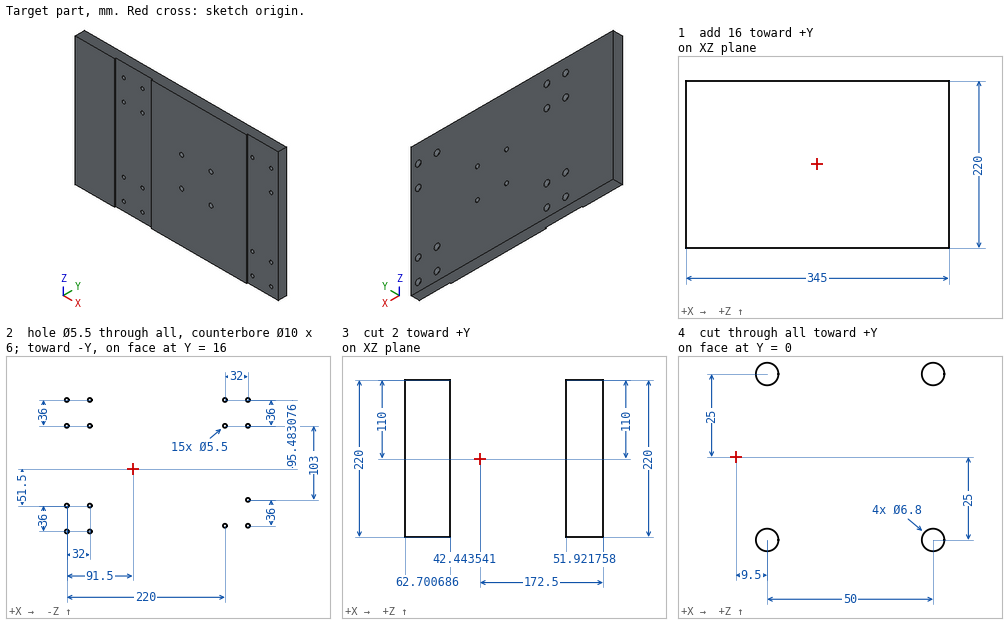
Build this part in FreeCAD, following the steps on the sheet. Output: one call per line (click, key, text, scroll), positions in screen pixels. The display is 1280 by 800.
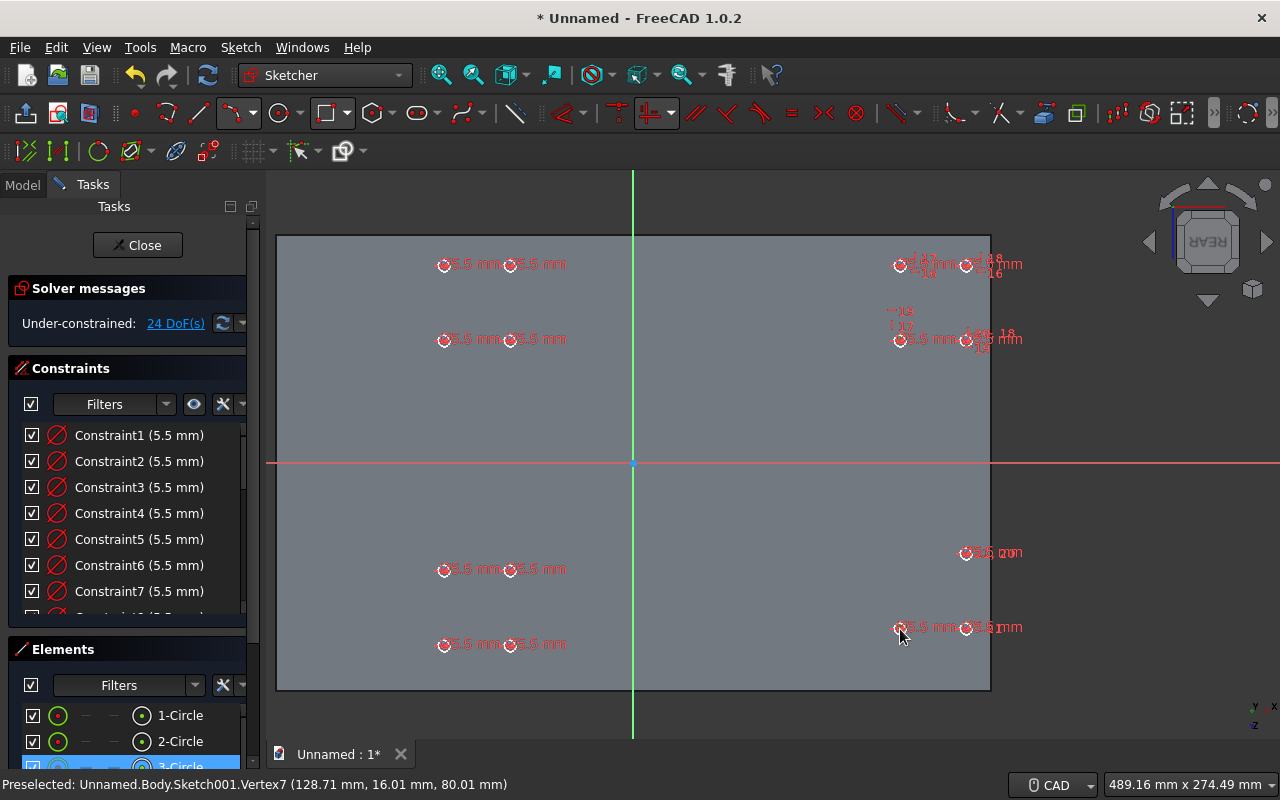
key(v)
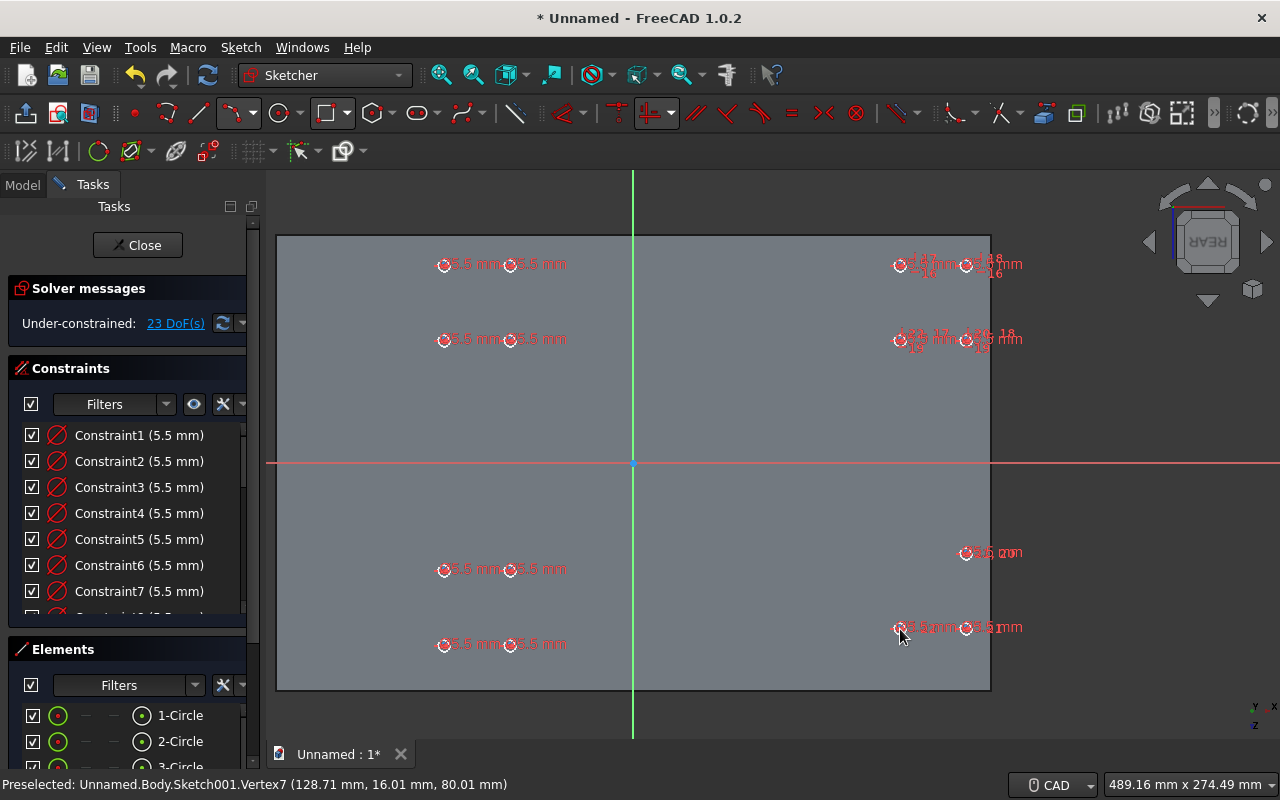
click(966, 629)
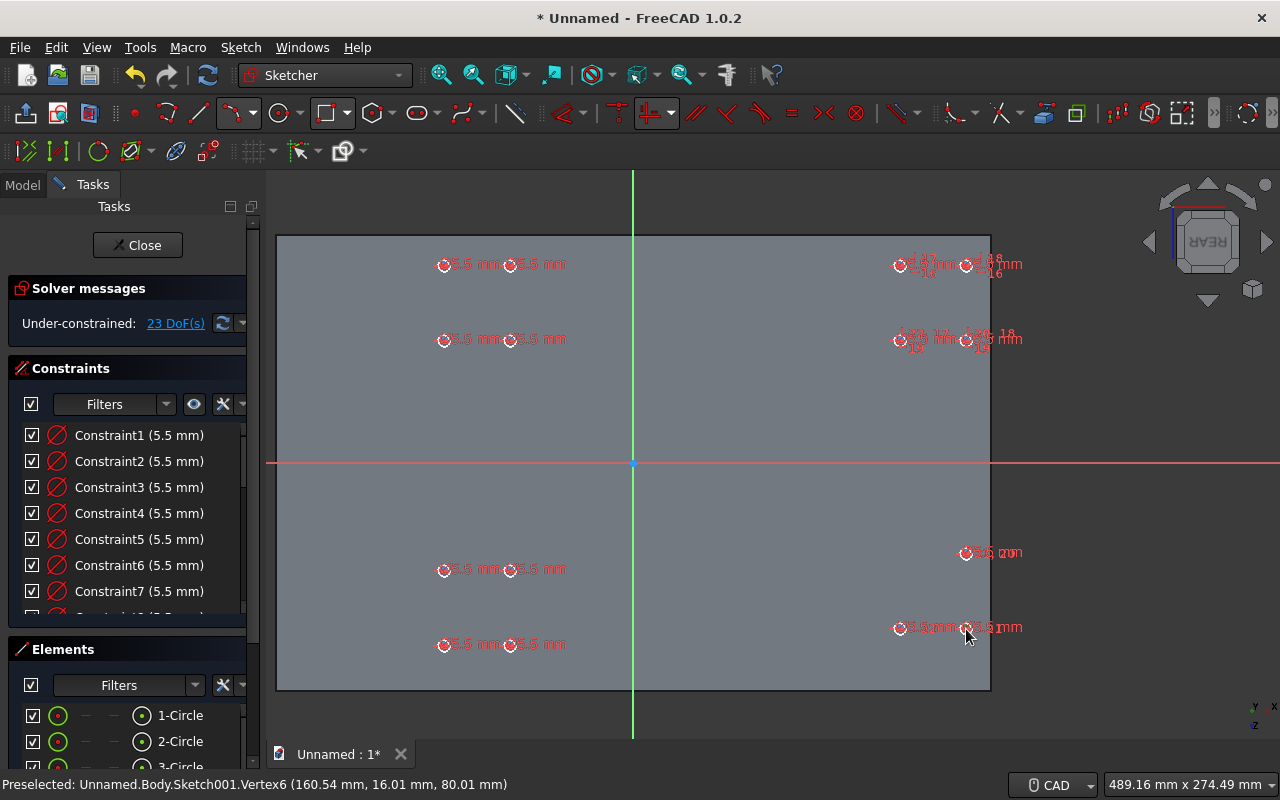
click(900, 629)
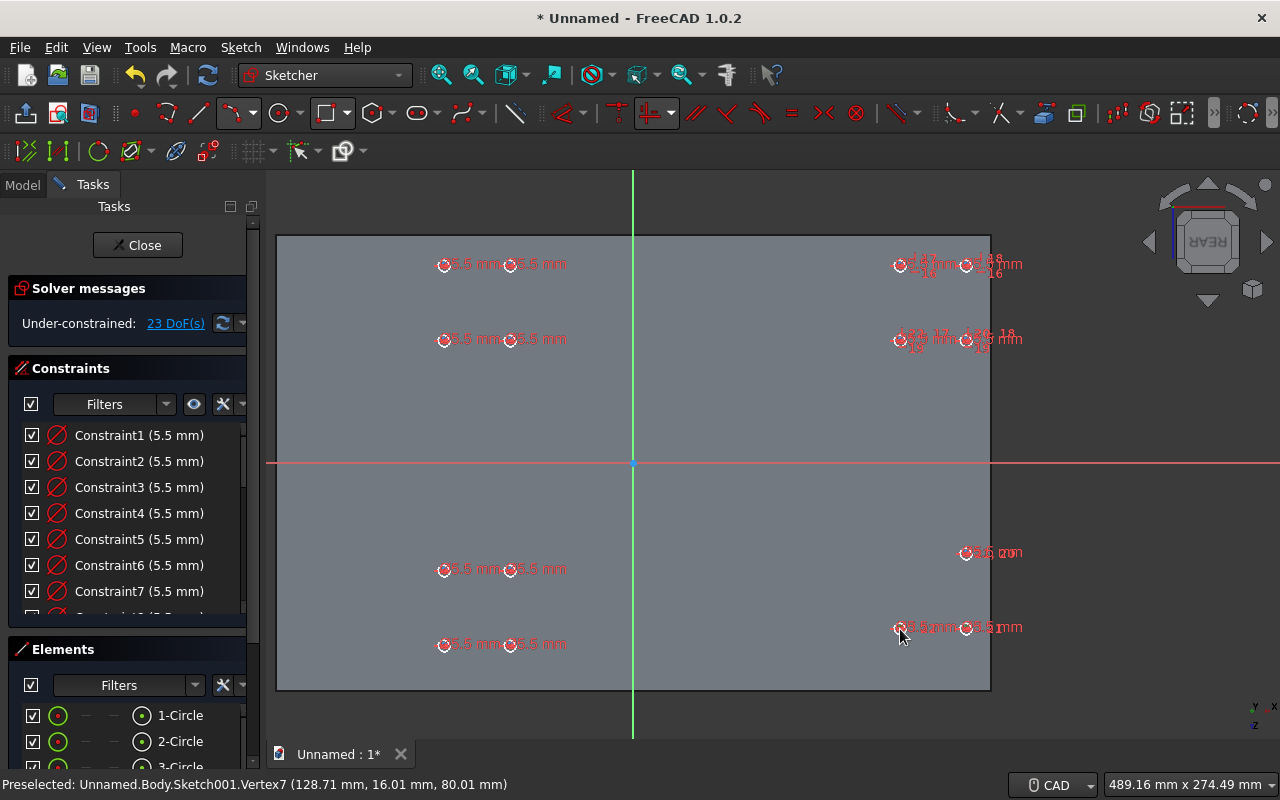
key(h)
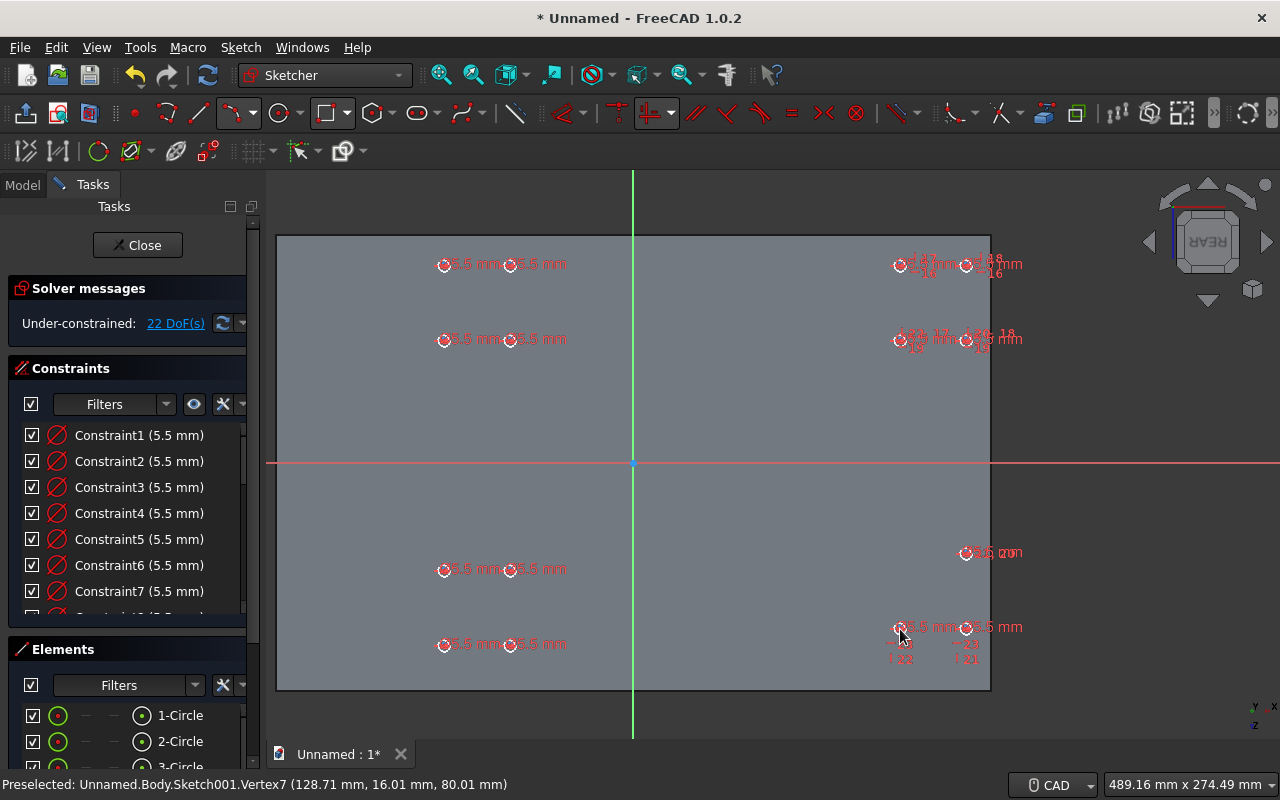
click(444, 571)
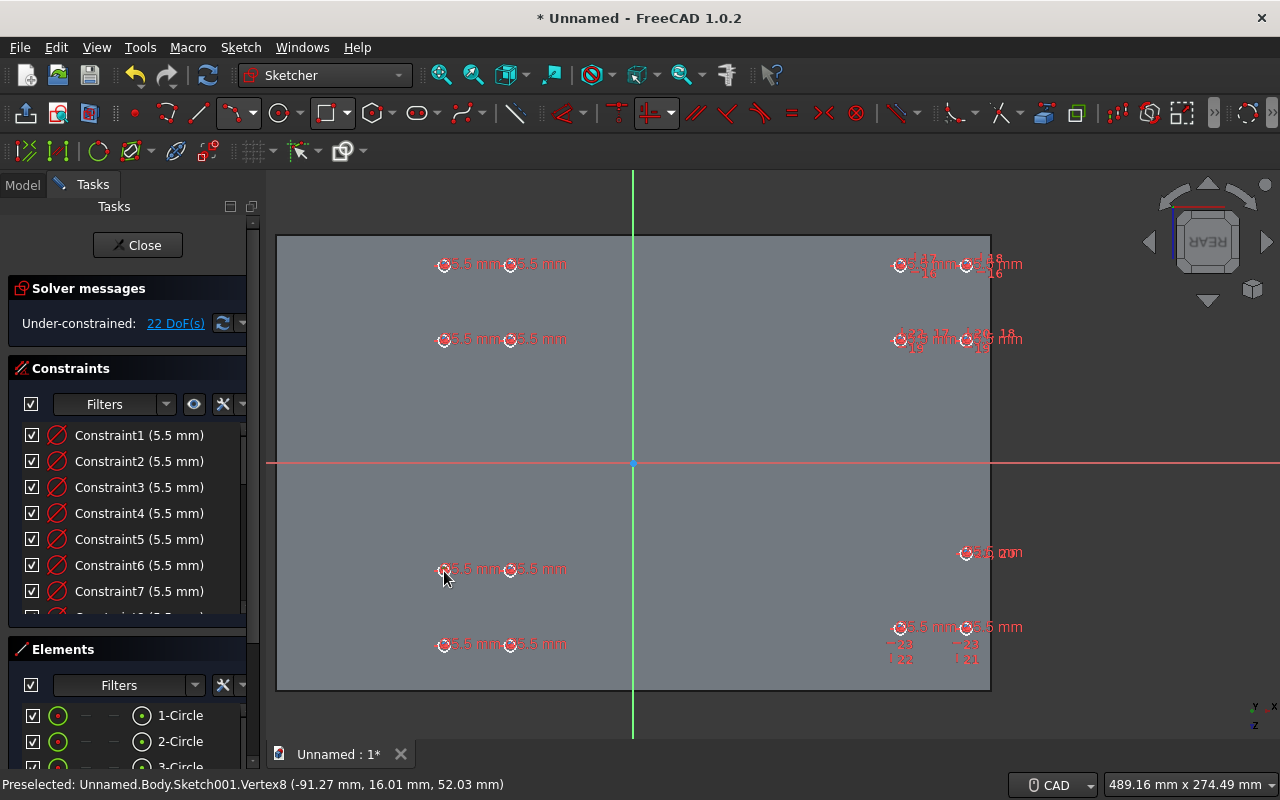
click(510, 571)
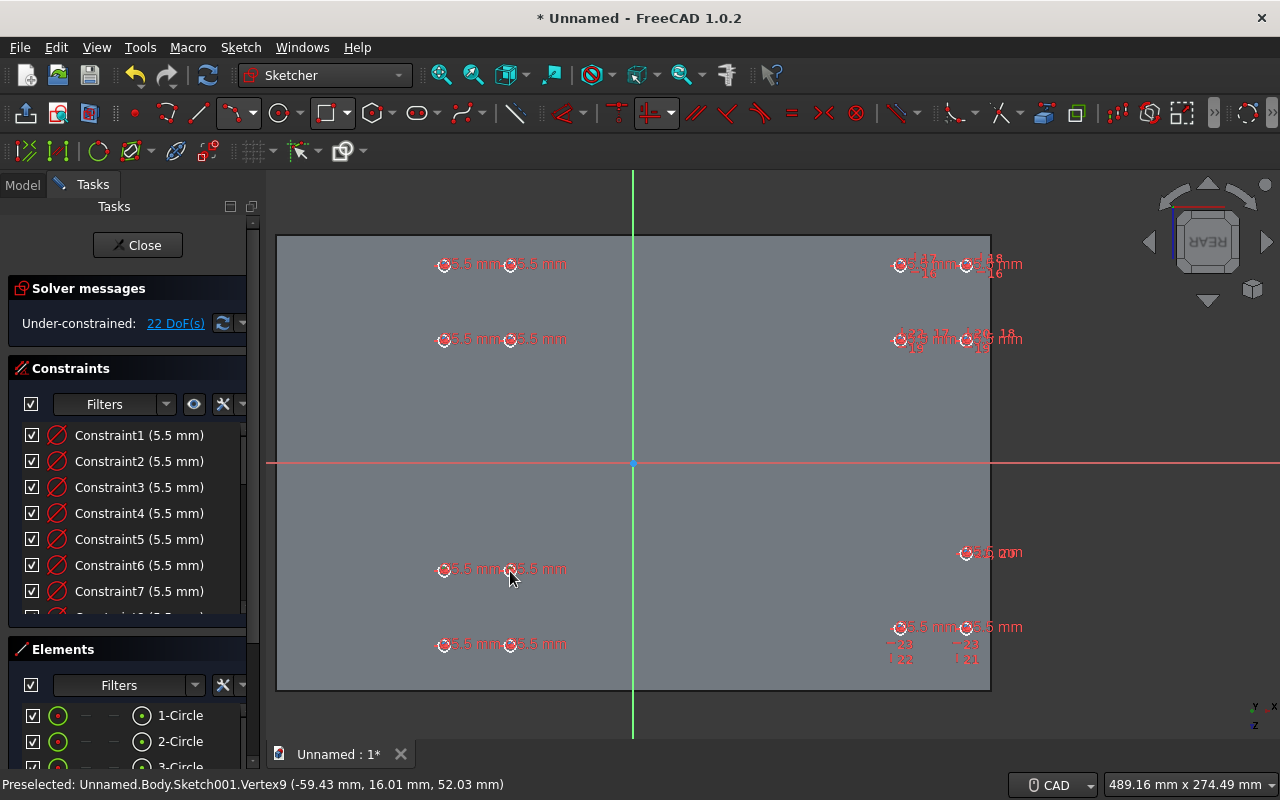
key(h)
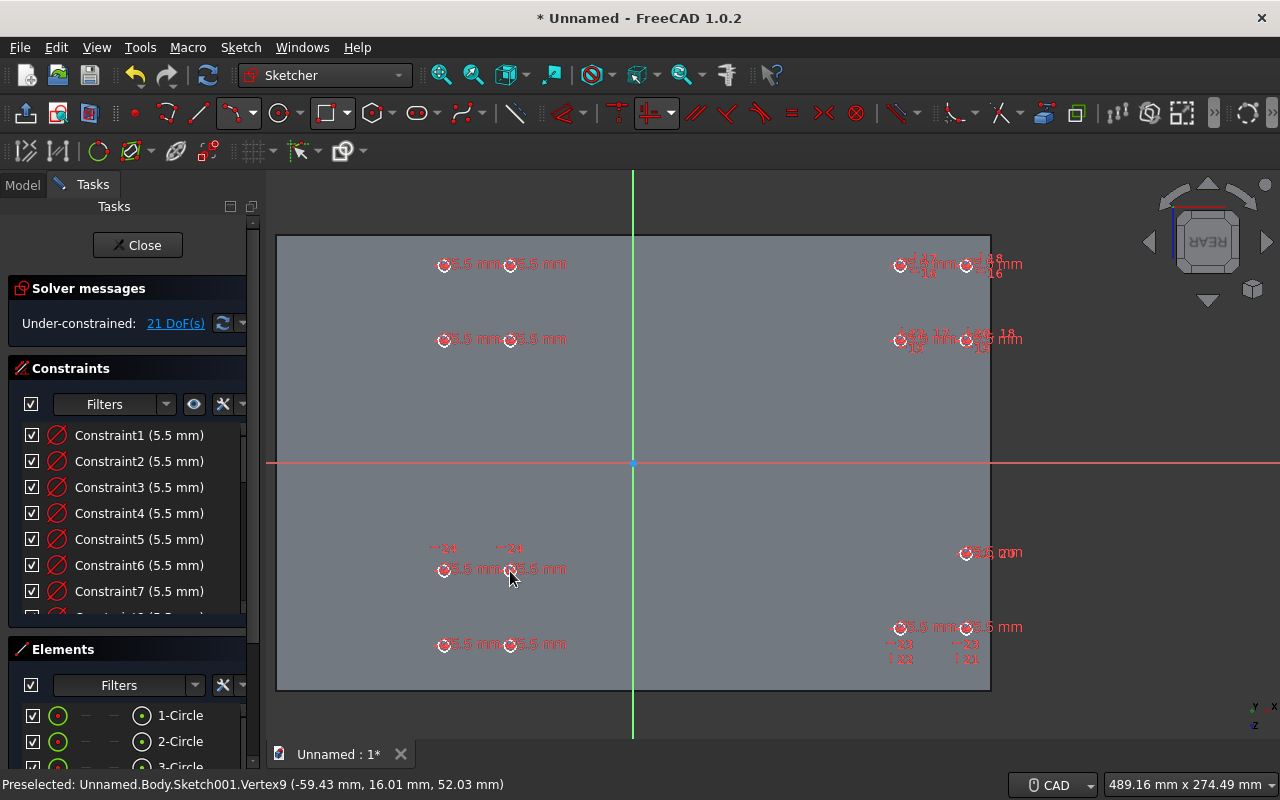
click(510, 571)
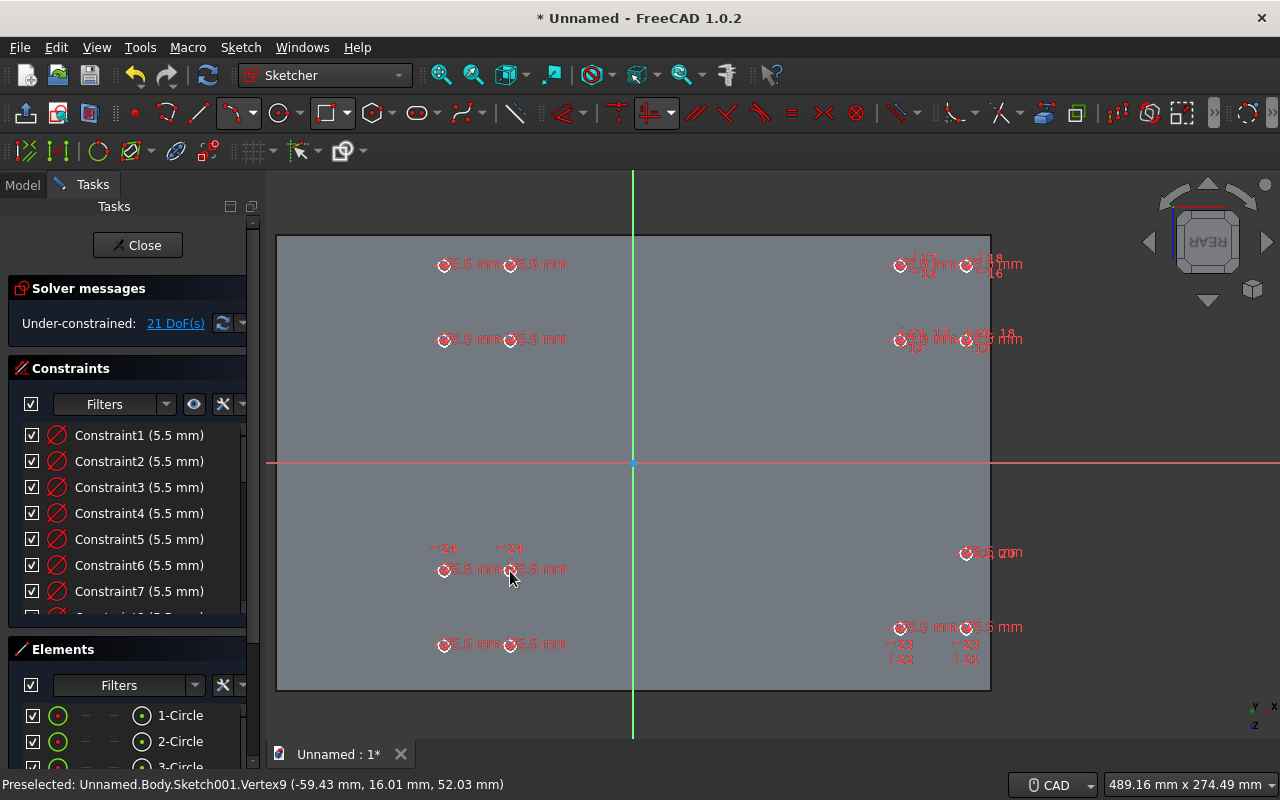
click(510, 646)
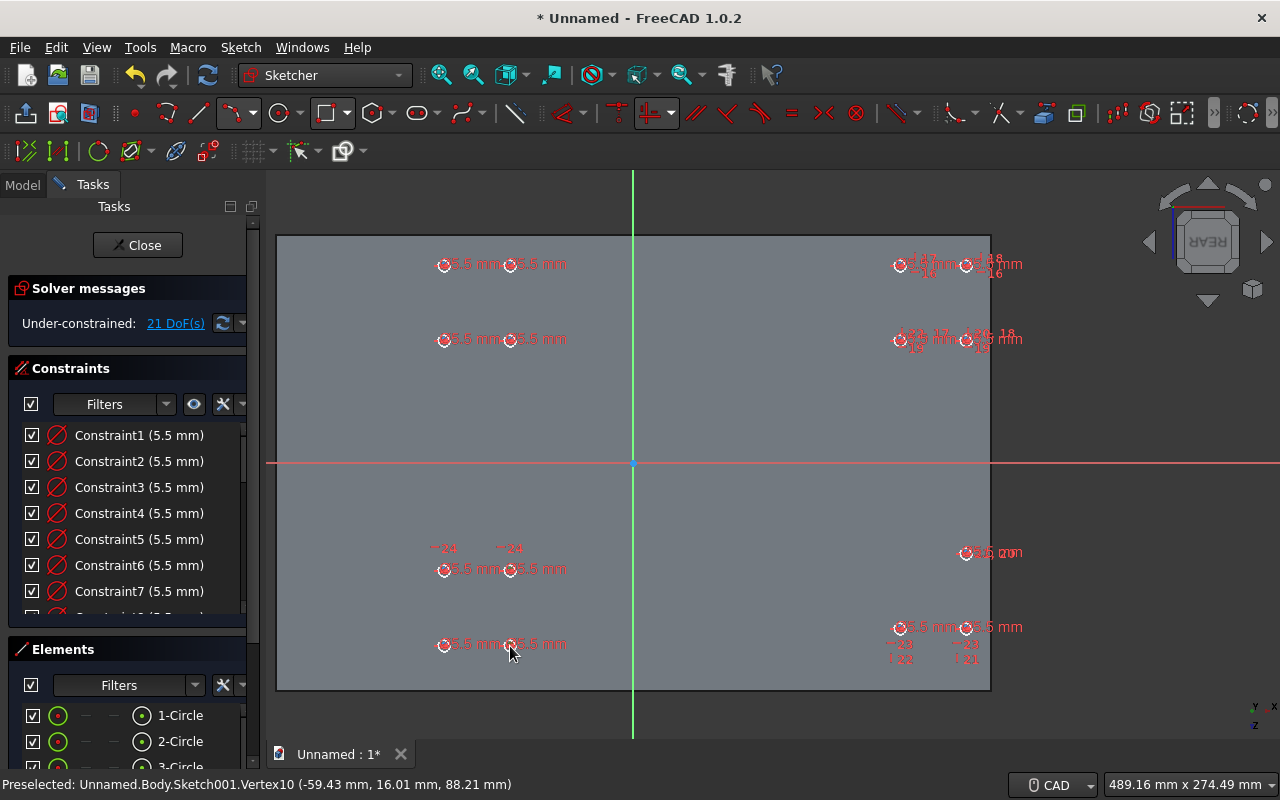
key(v)